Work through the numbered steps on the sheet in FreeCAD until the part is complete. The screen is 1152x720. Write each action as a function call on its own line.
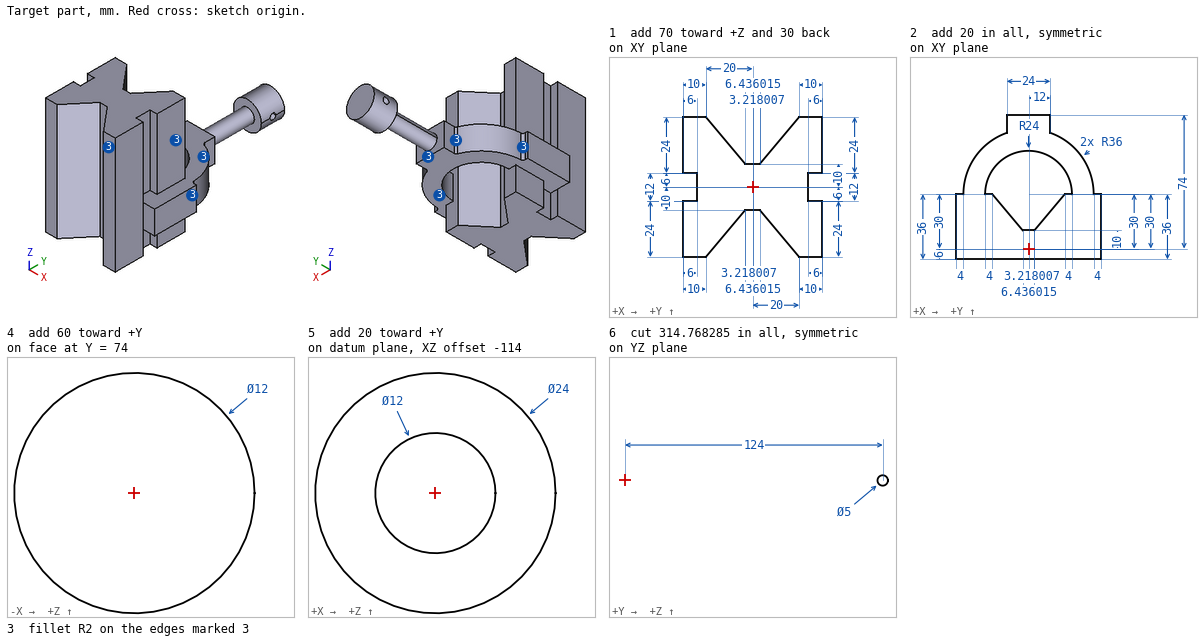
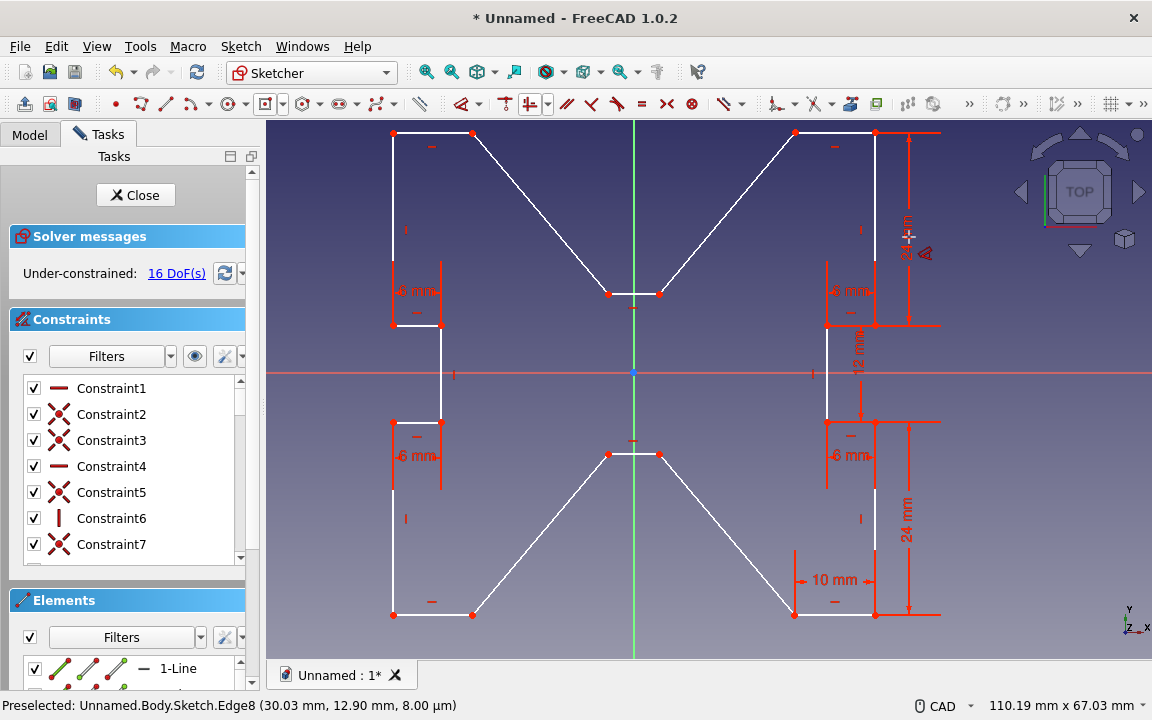
scroll(654, 424, down, 2)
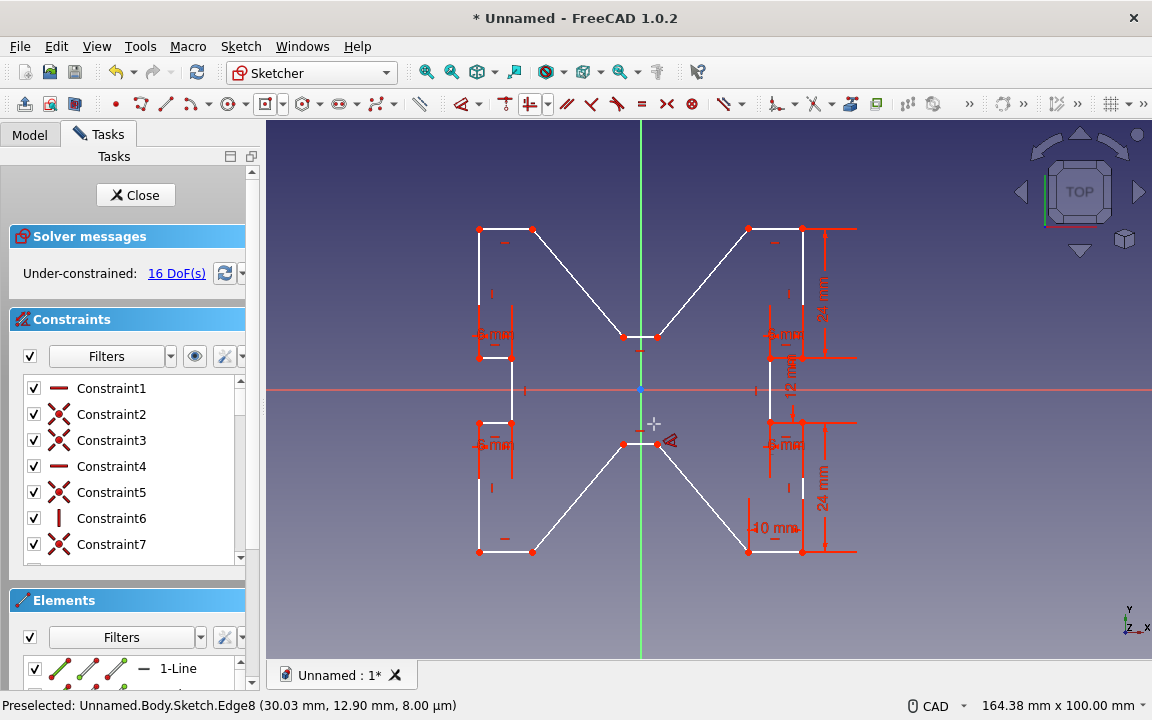
click(786, 229)
click(776, 195)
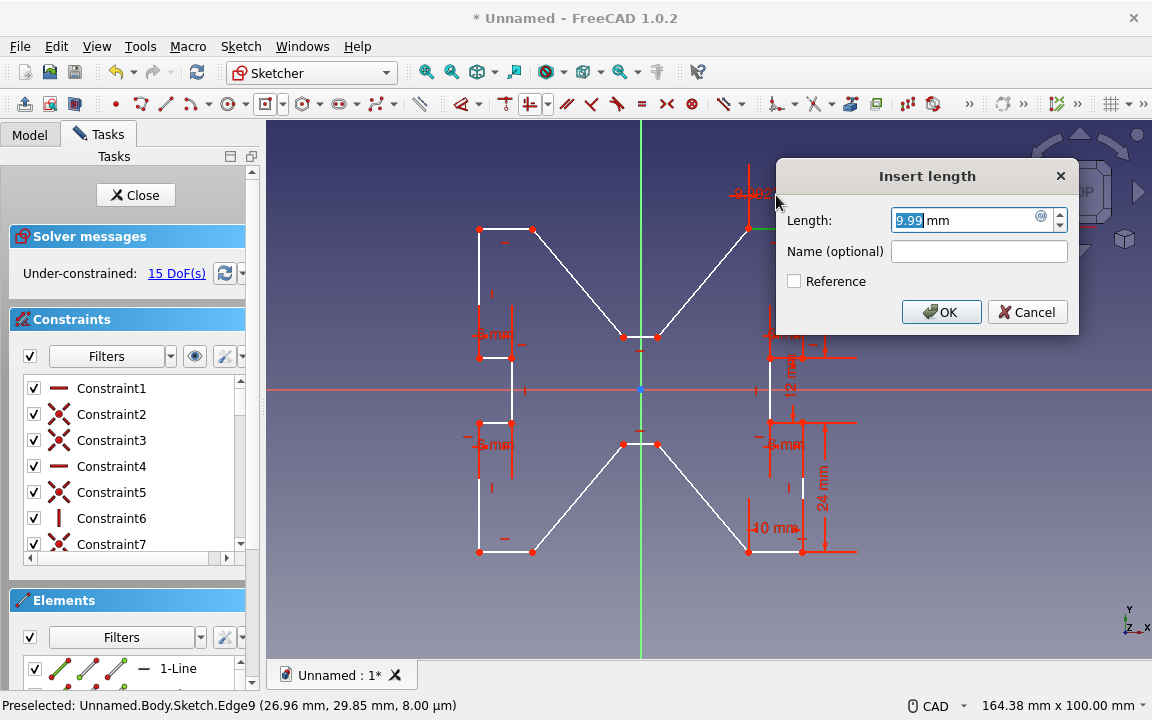
text(10)
key(Return)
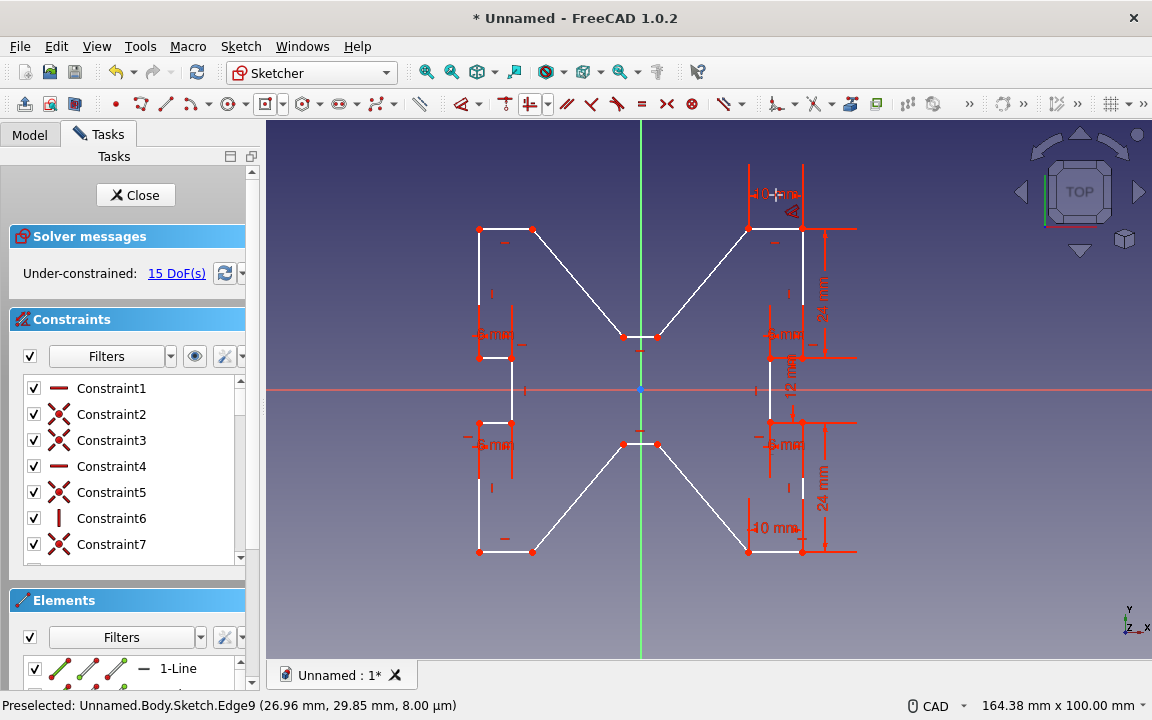
click(517, 229)
click(506, 195)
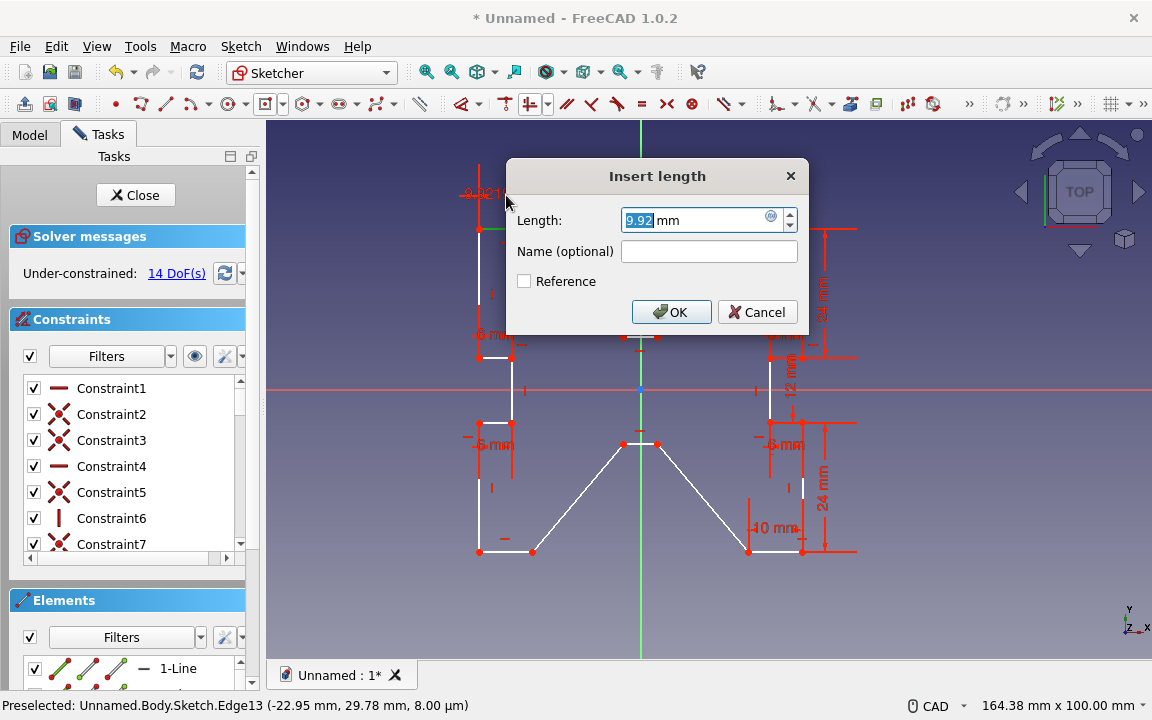
text(10)
key(Return)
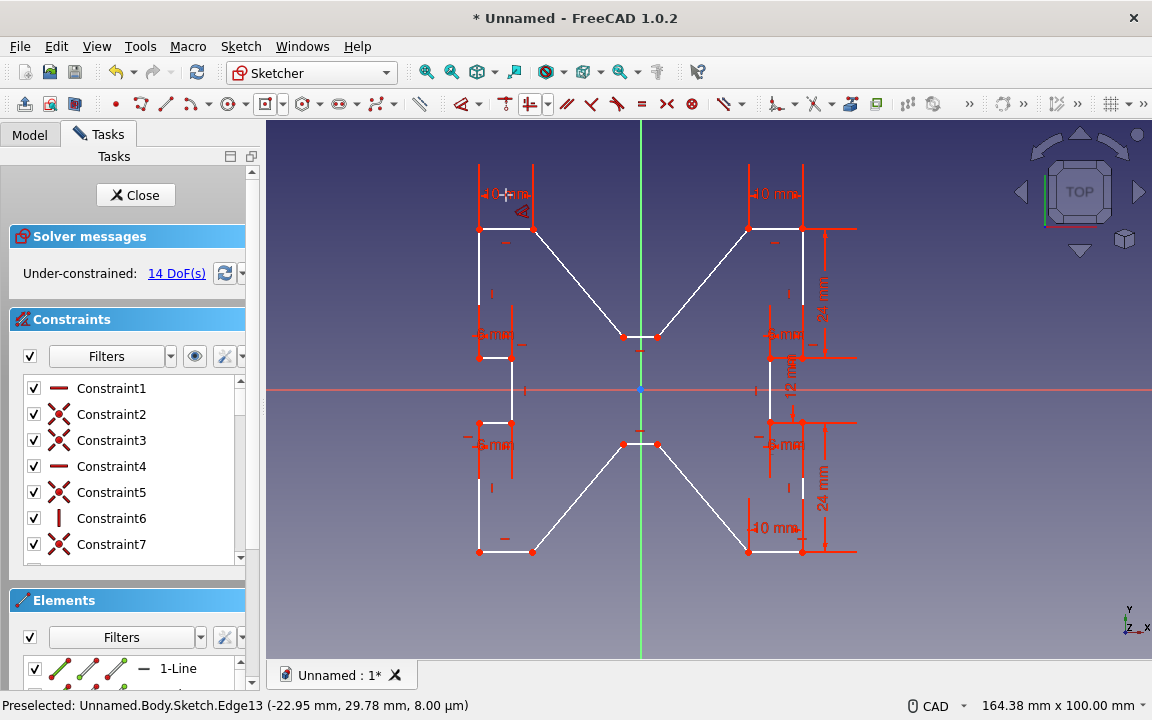
click(479, 268)
click(445, 294)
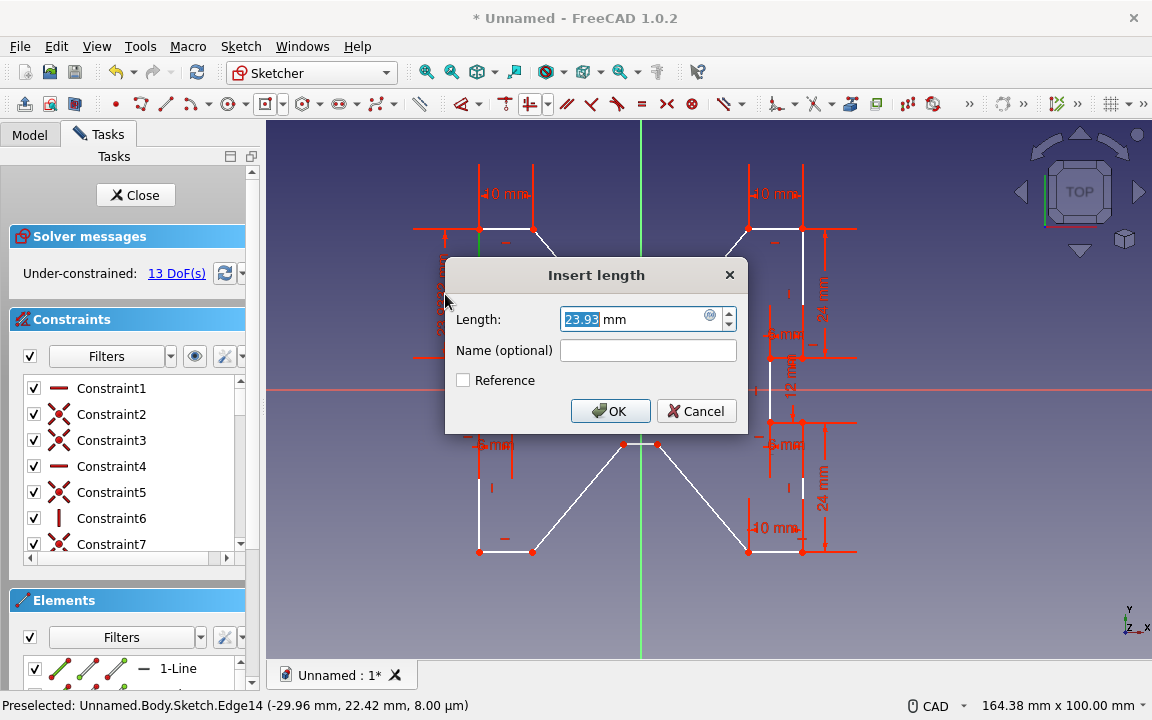
text(24)
key(Return)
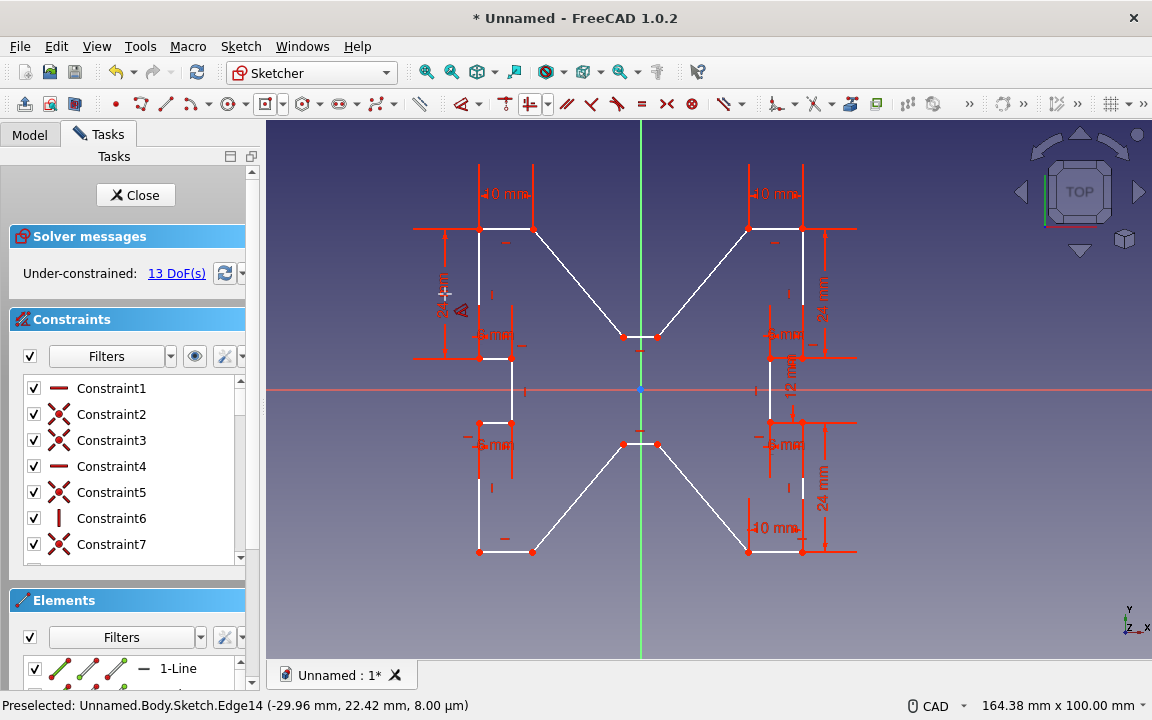
click(512, 378)
click(478, 376)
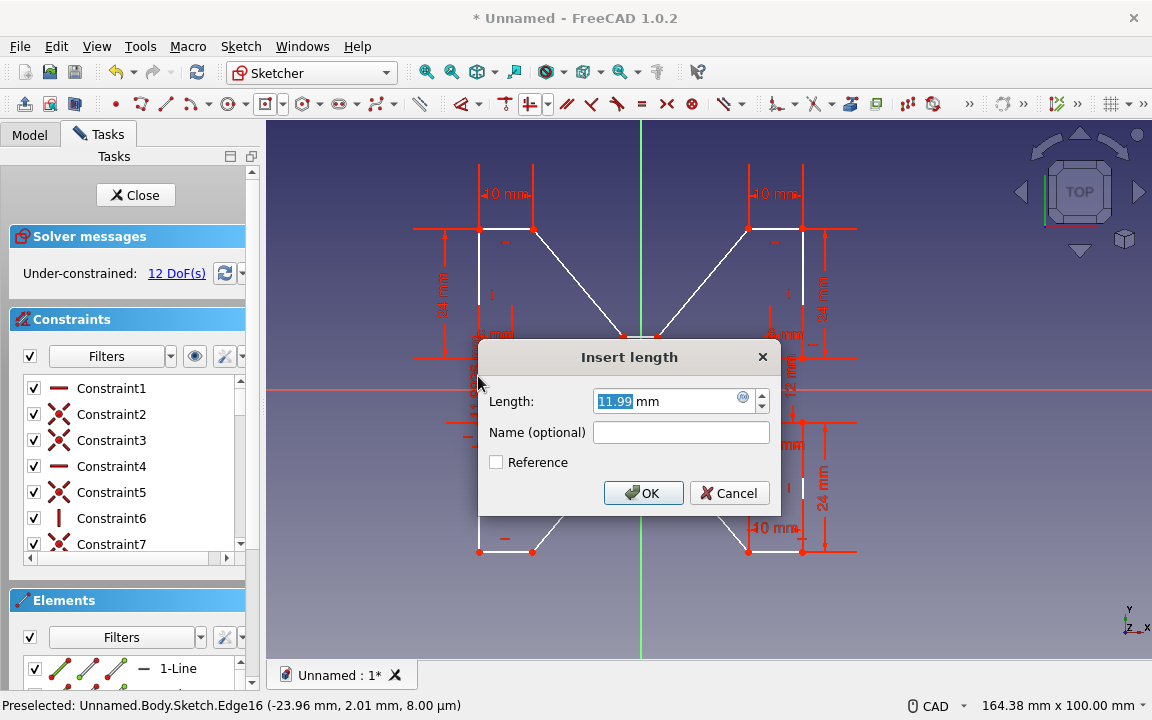
text(12)
key(Return)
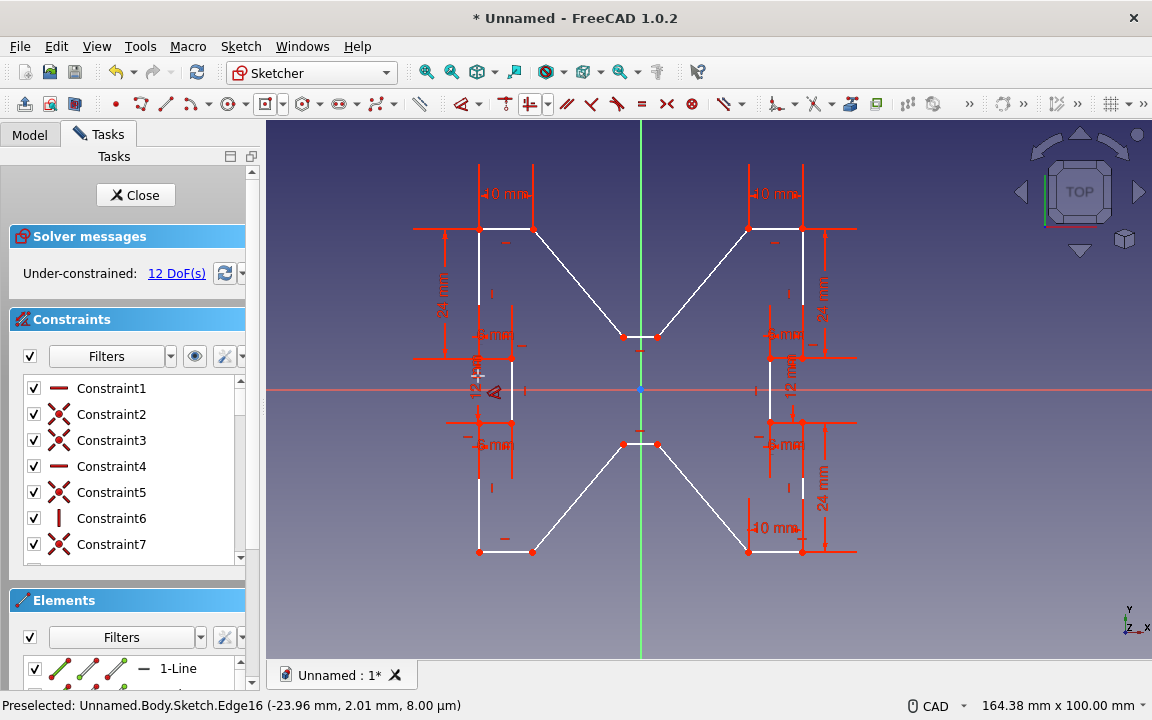
click(479, 462)
click(445, 488)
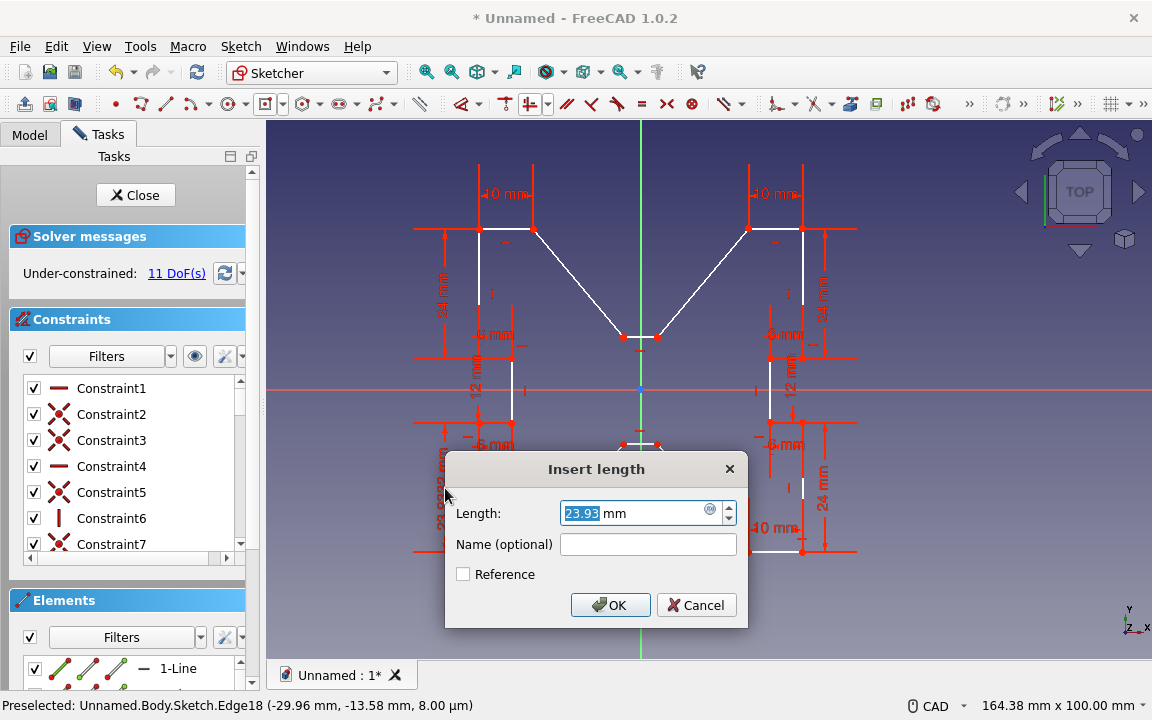
text(24)
key(Return)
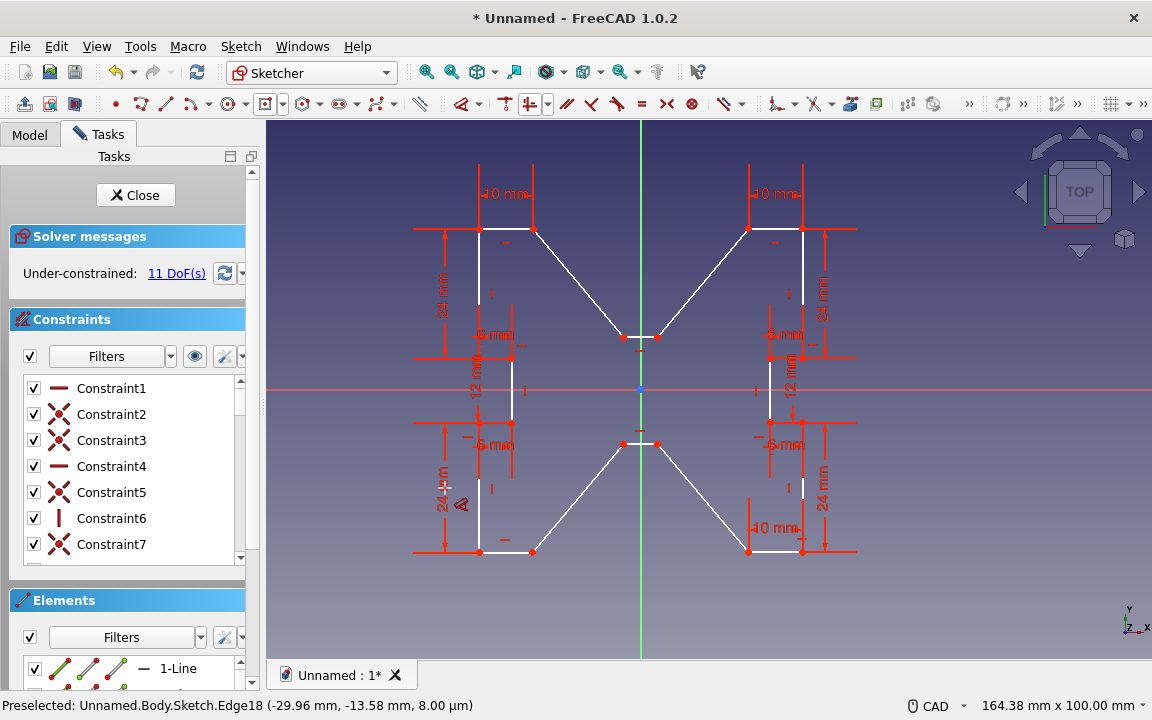
click(495, 553)
click(506, 587)